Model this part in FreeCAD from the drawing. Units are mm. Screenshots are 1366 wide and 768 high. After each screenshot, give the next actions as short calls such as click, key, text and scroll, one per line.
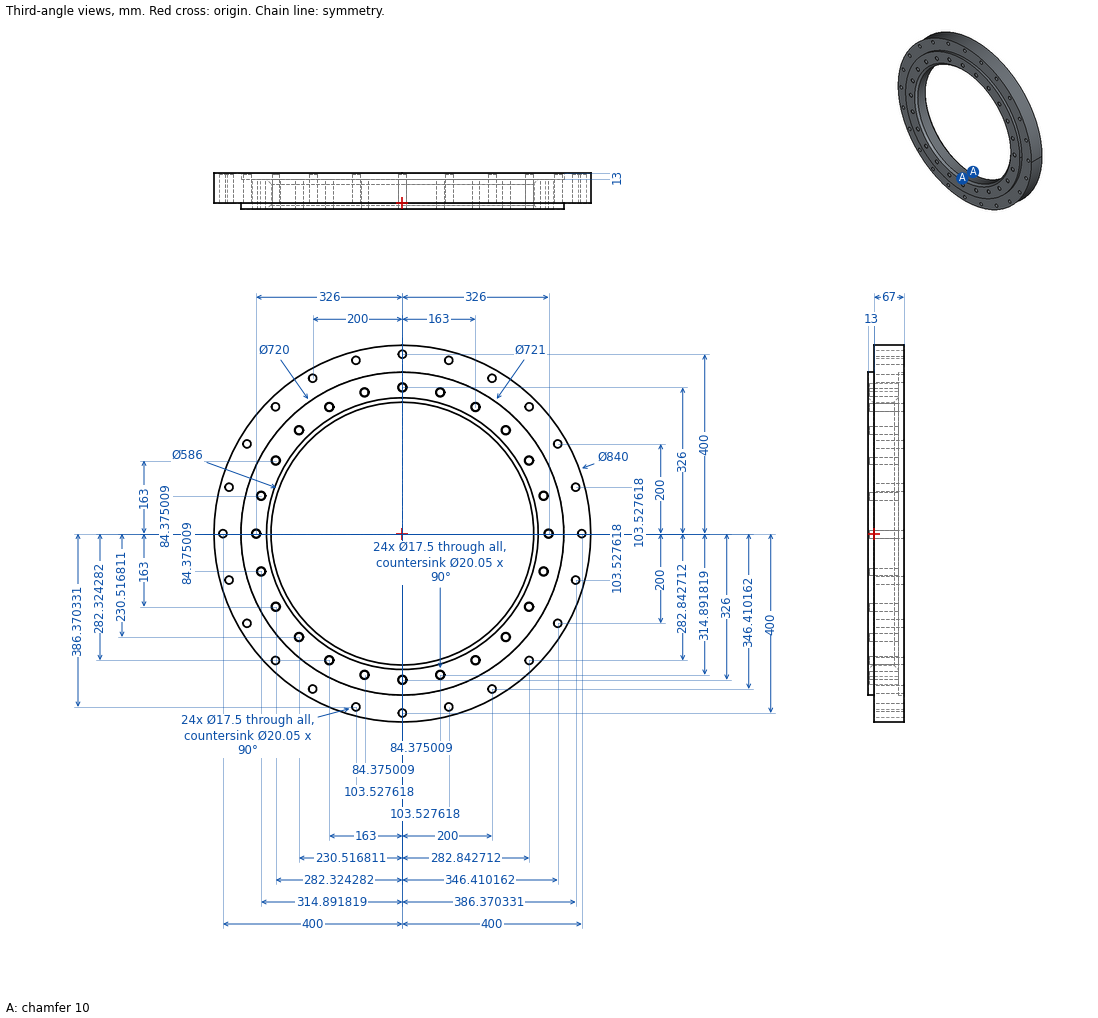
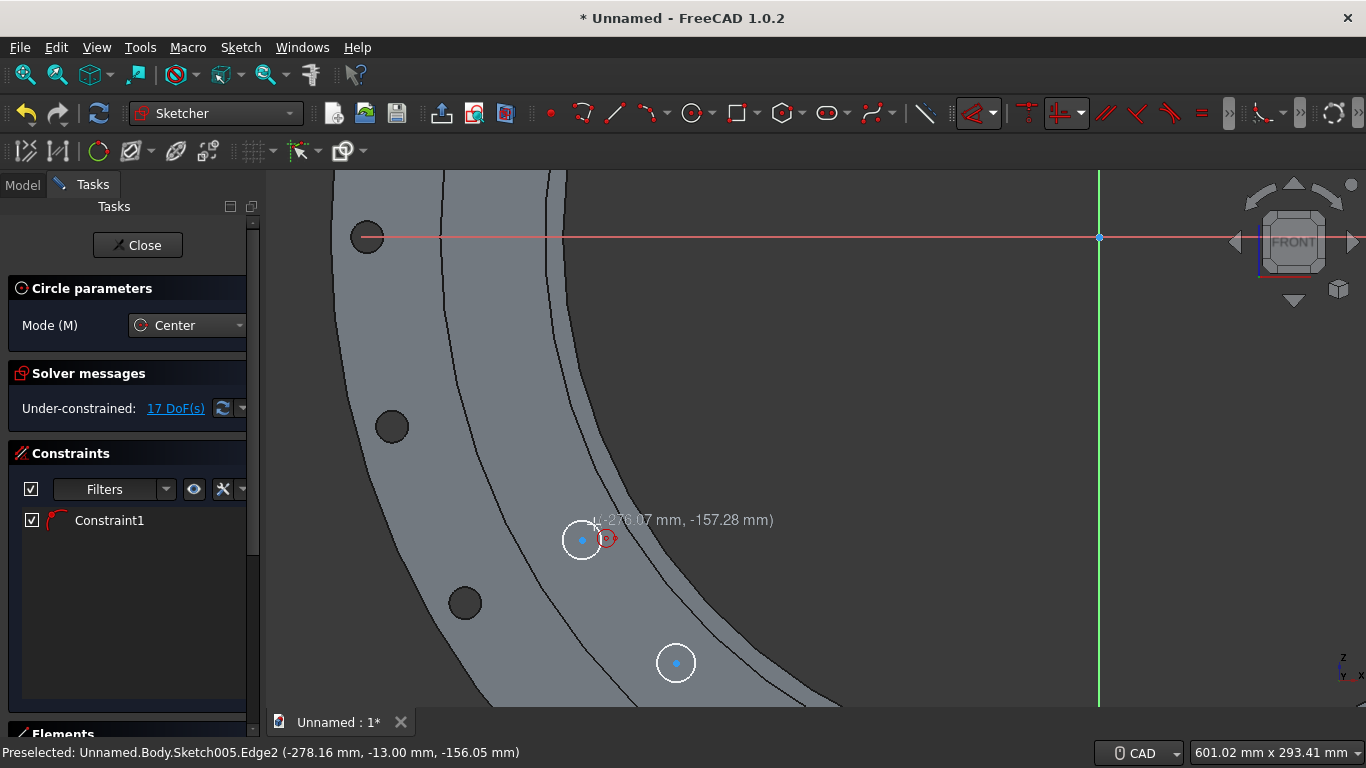
scroll(523, 392, up, 2)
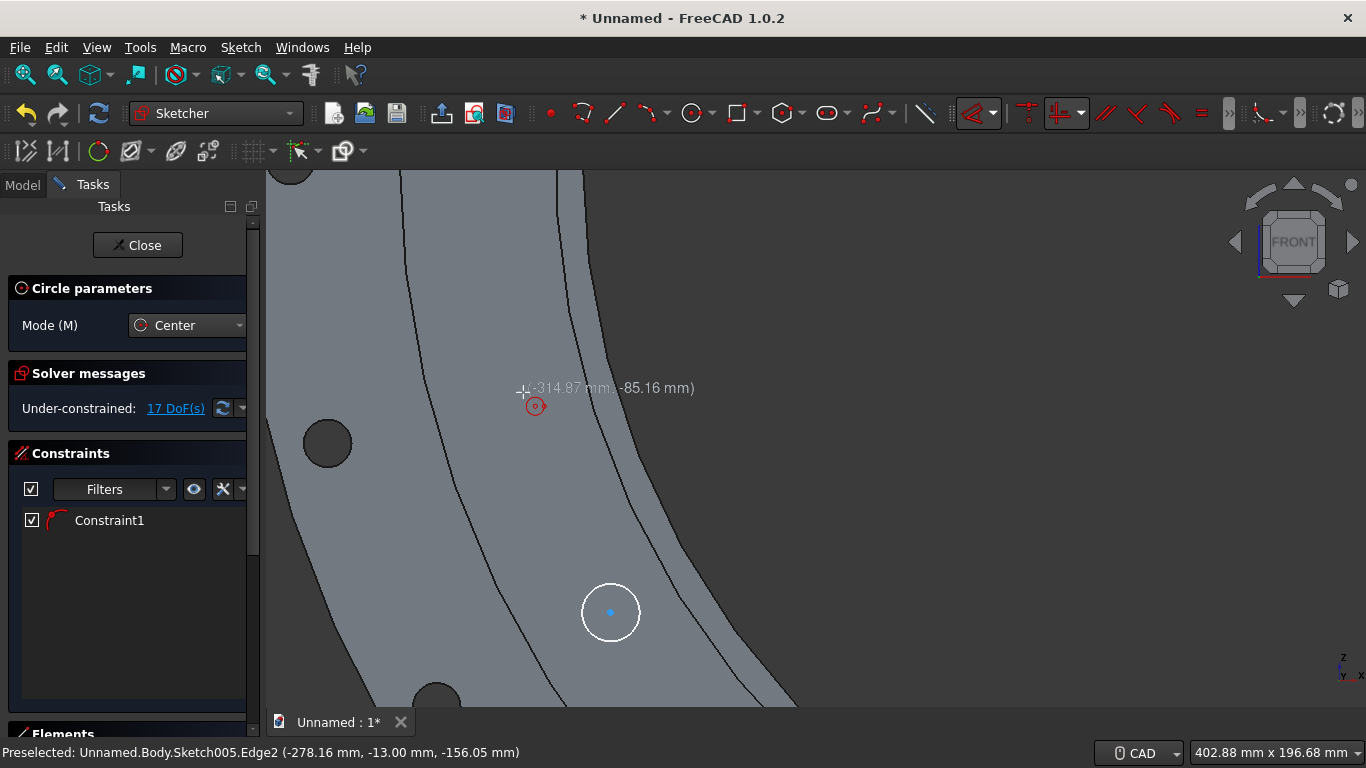
scroll(587, 509, down, 8)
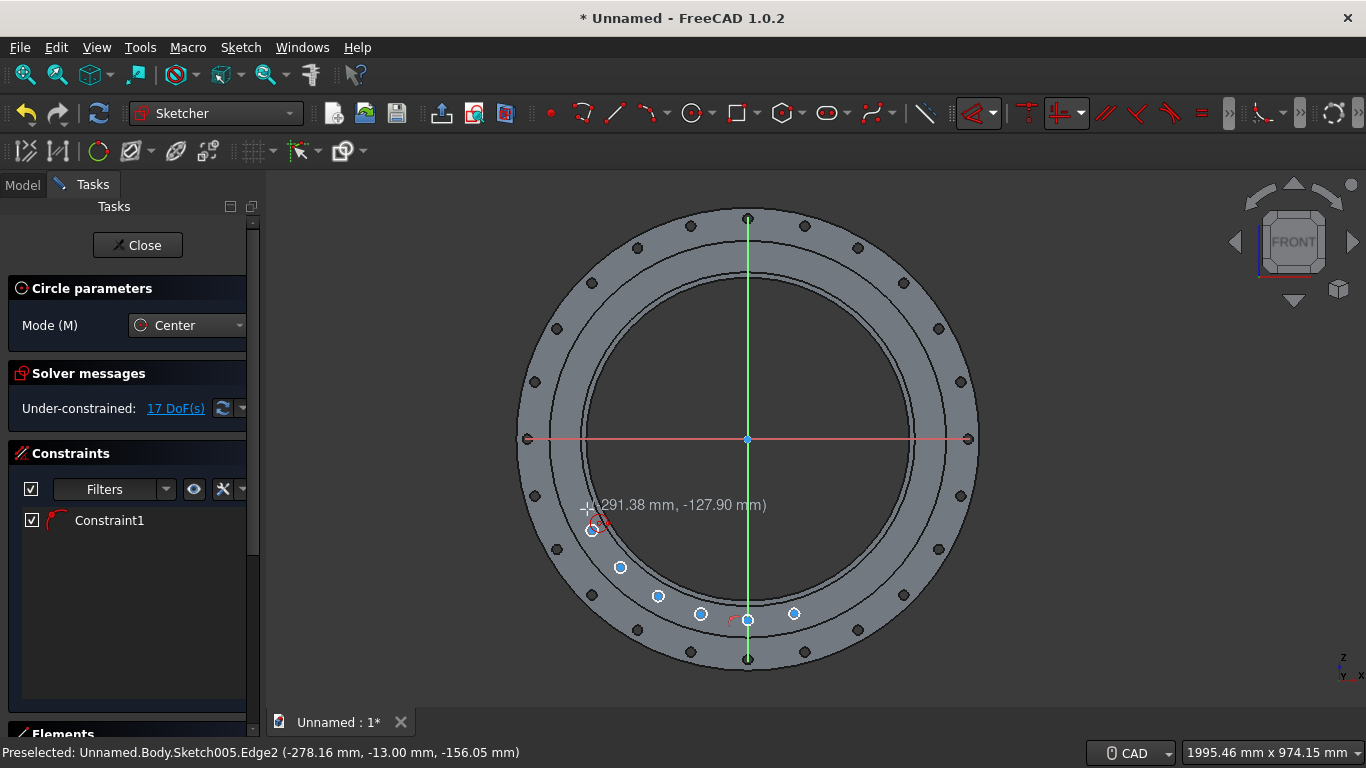
click(574, 486)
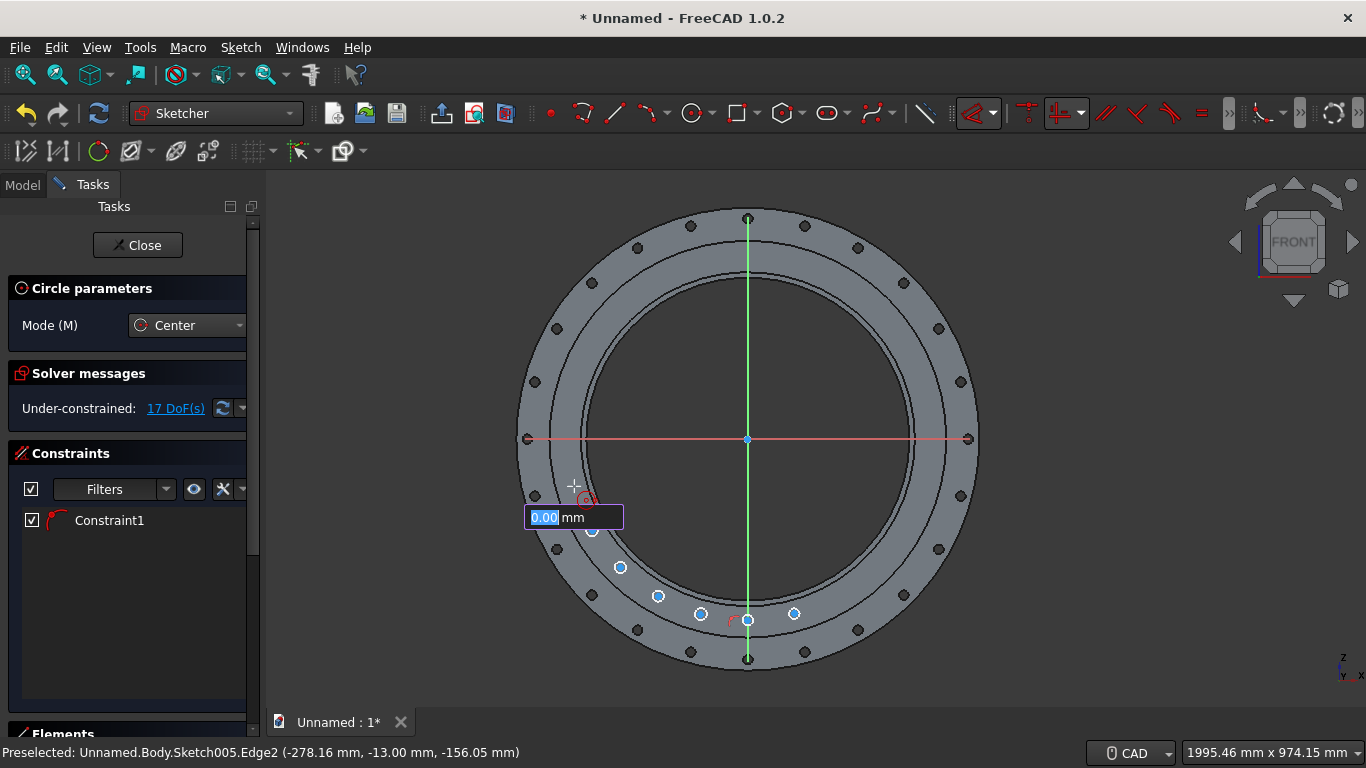
scroll(578, 482, up, 6)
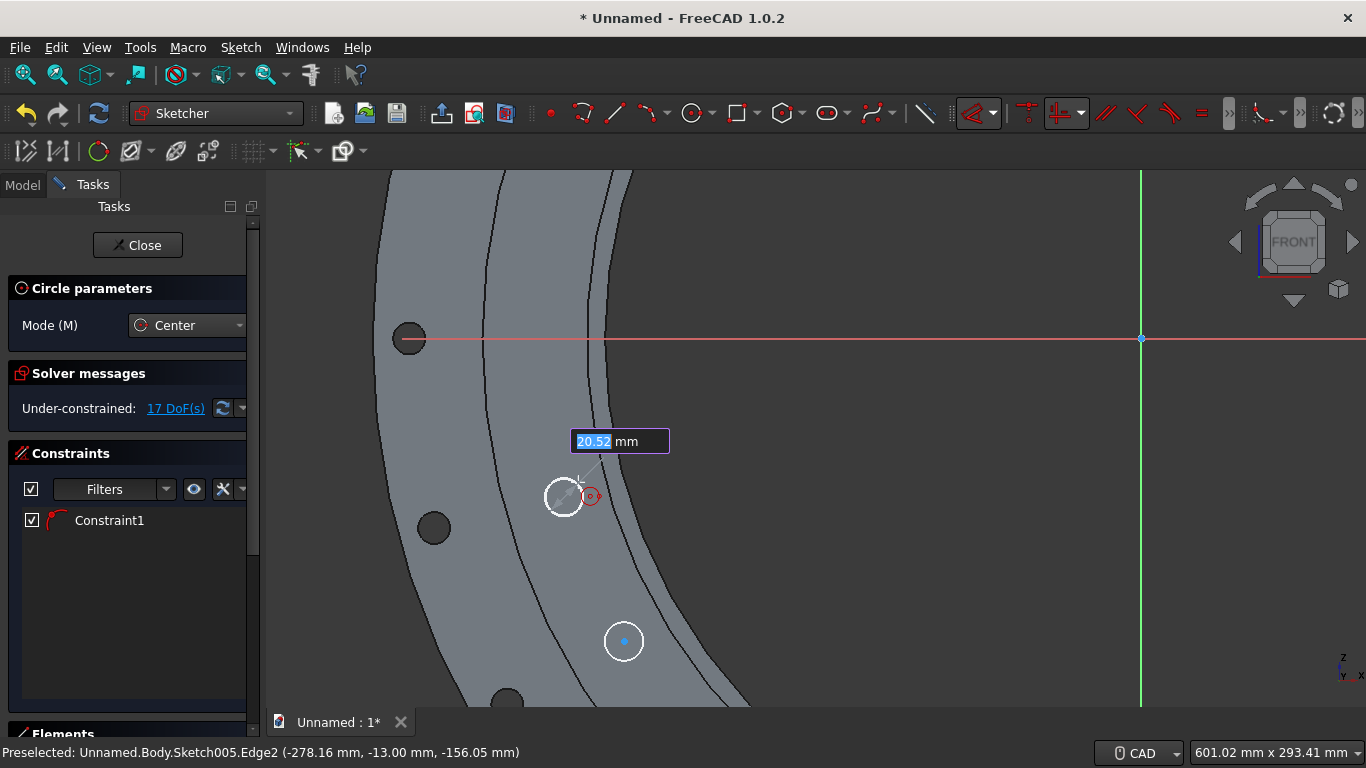
click(576, 482)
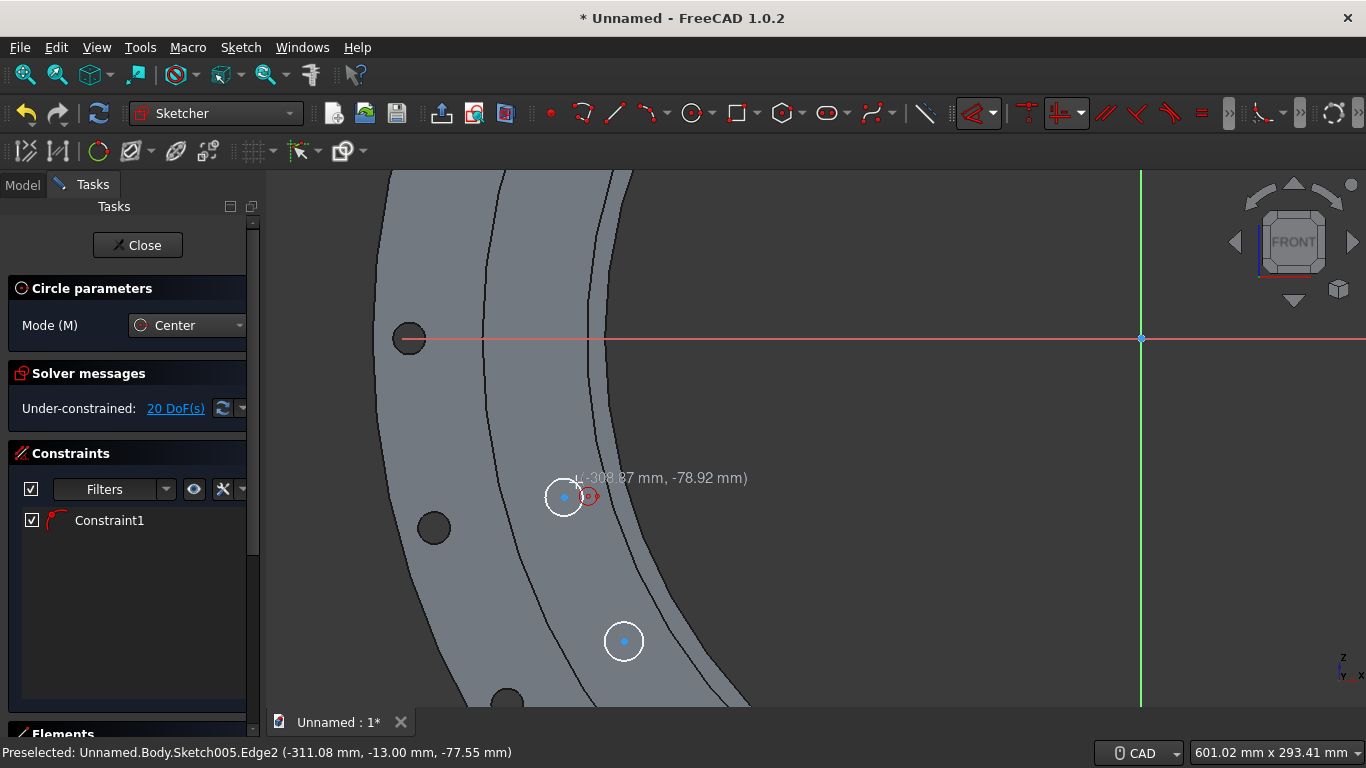
scroll(545, 339, up, 2)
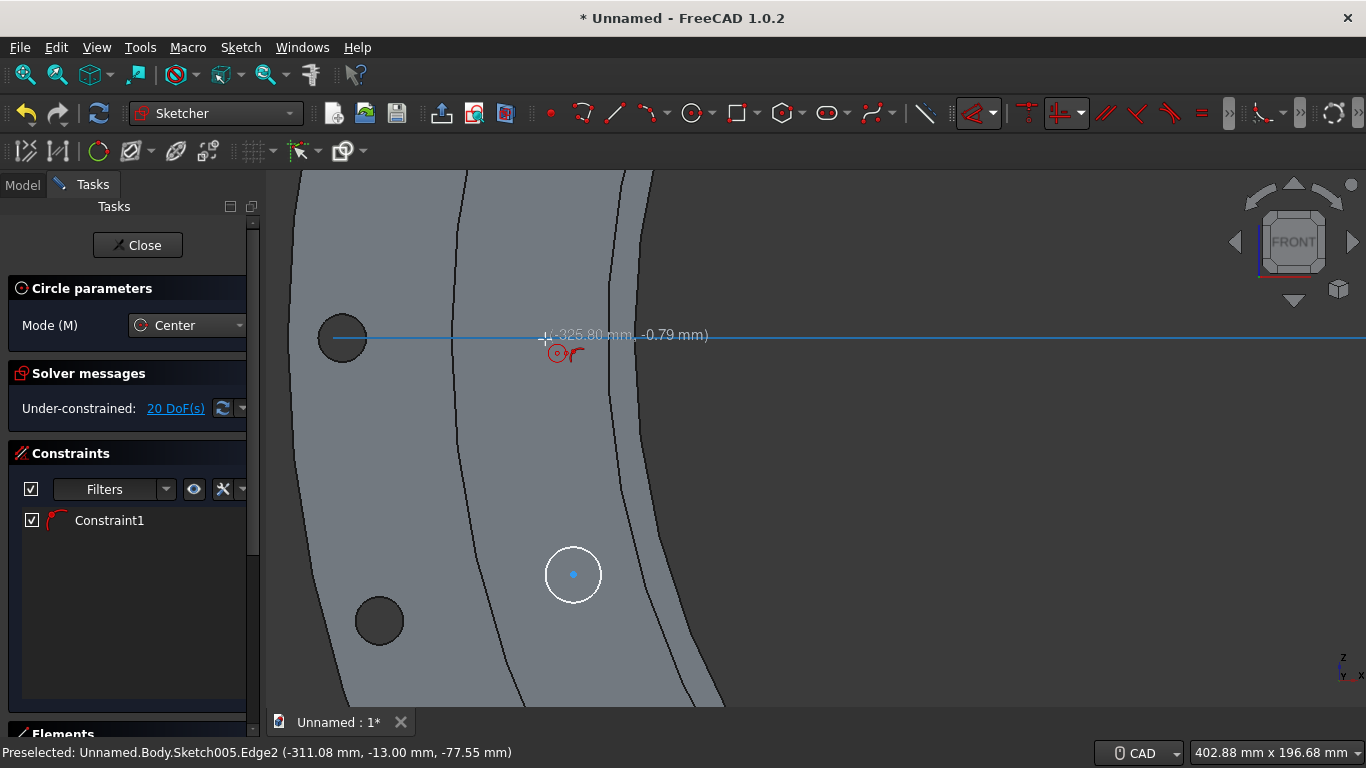
scroll(574, 464, down, 8)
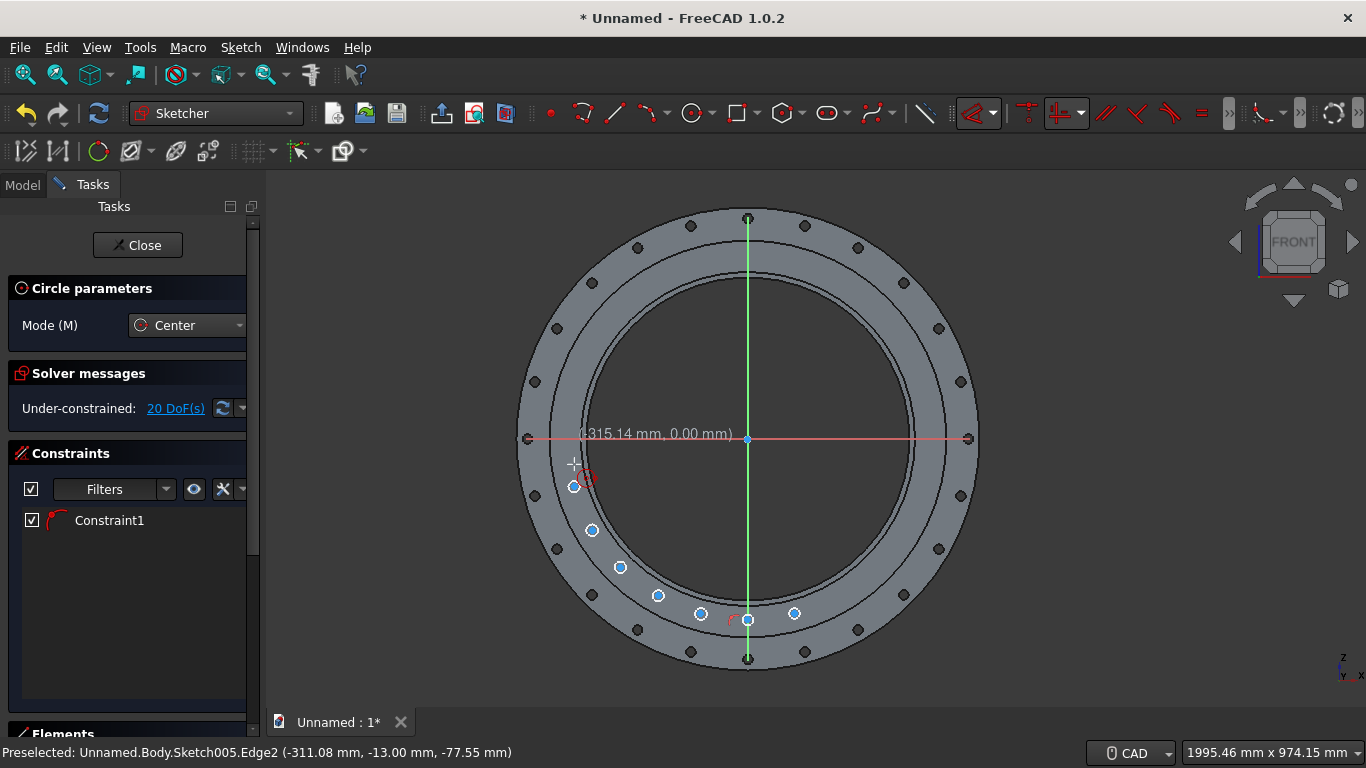
click(568, 439)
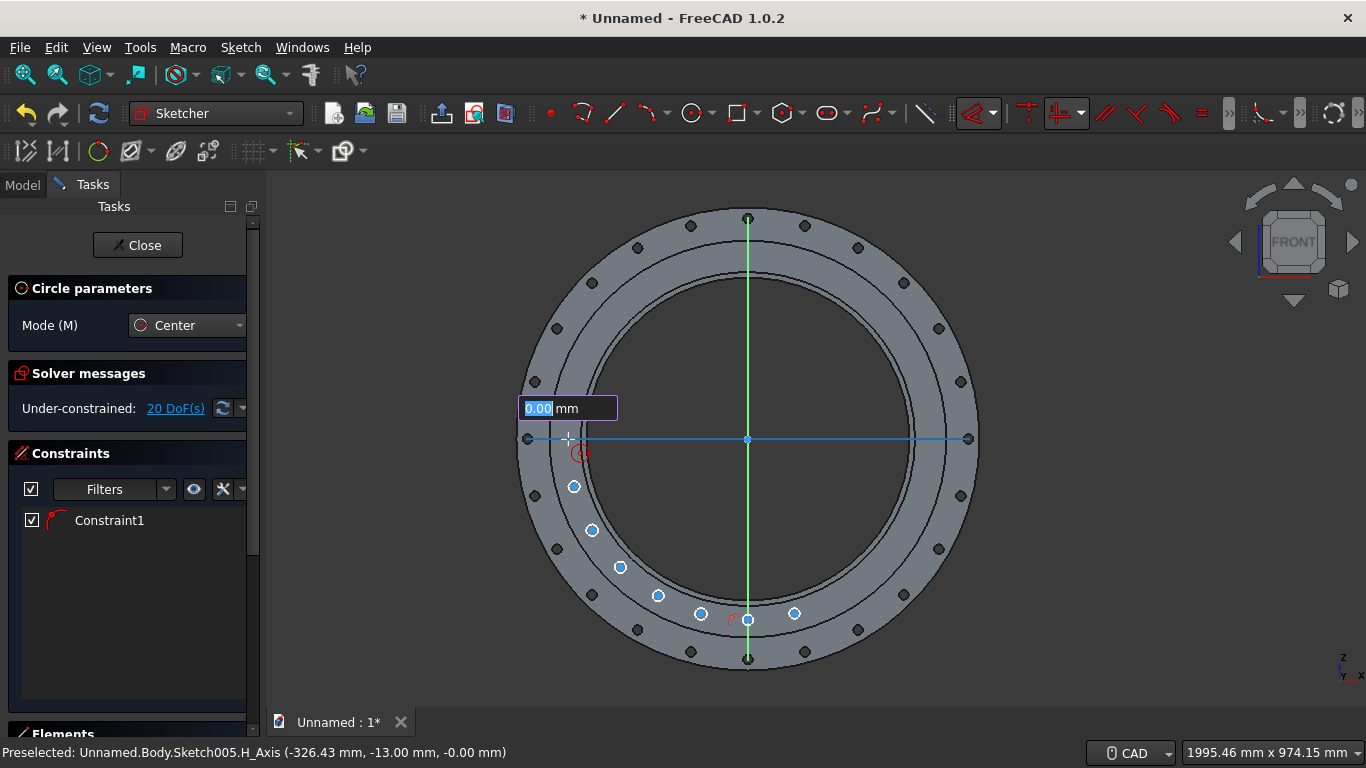
scroll(570, 435, up, 7)